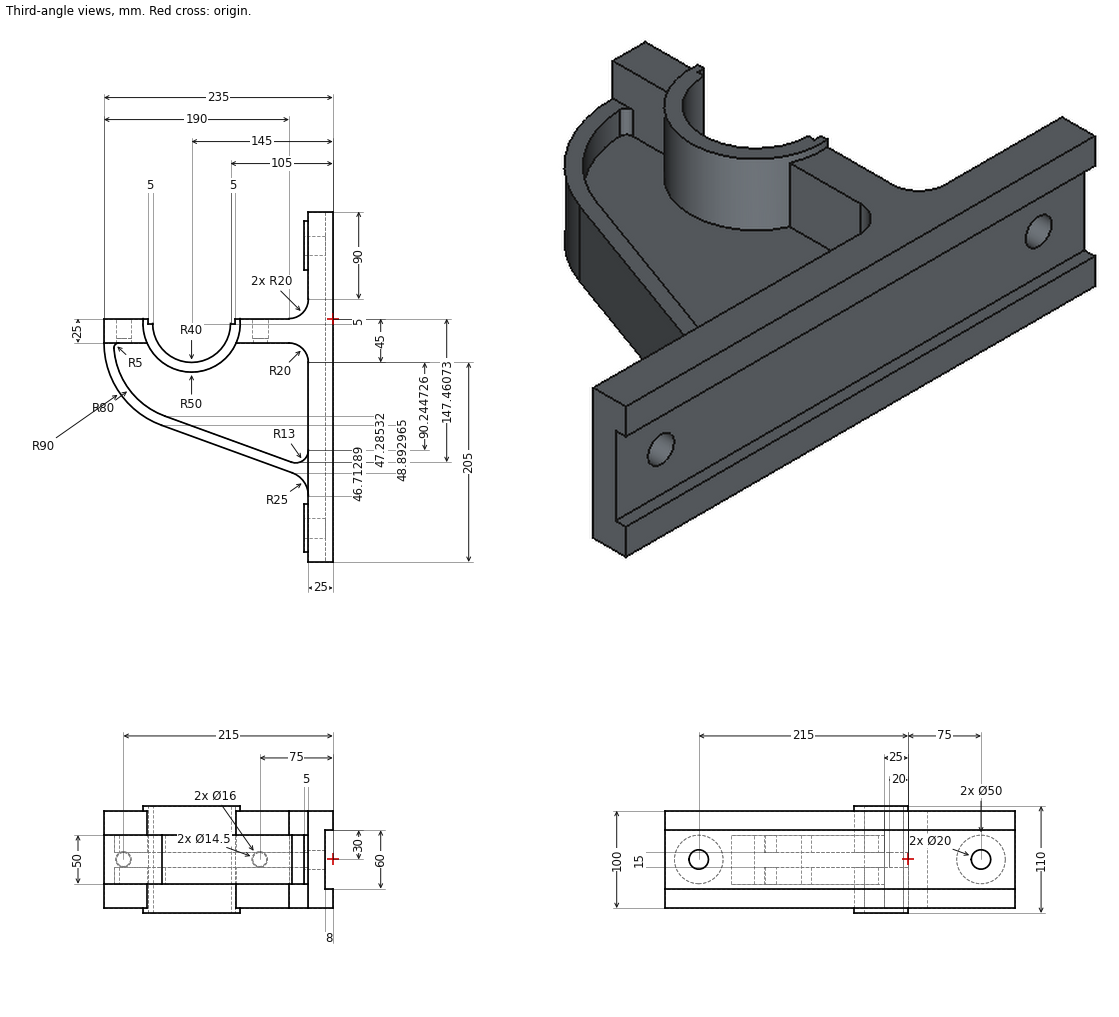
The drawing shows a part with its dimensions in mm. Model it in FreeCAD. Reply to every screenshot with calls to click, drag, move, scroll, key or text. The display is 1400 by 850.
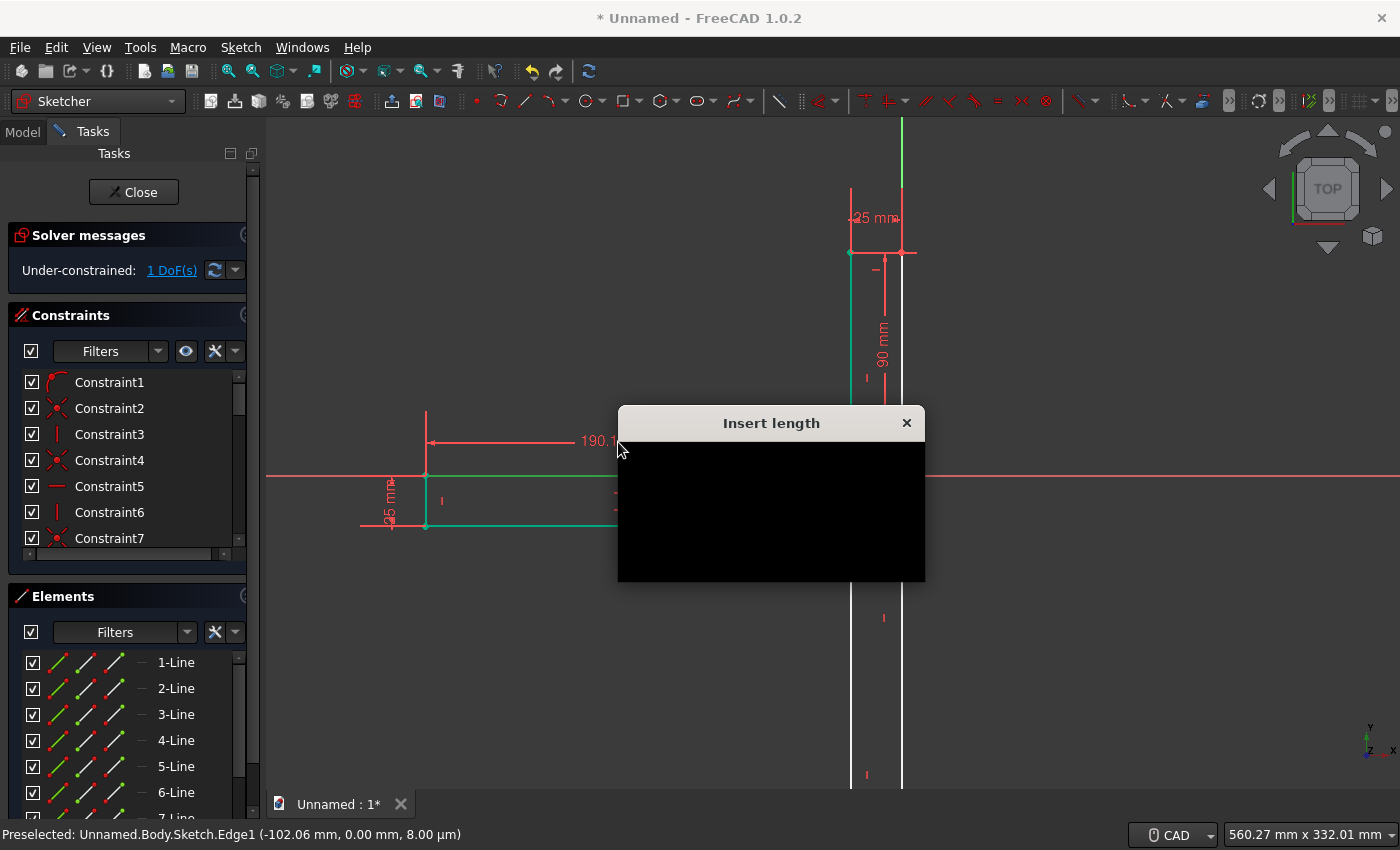
text(190)
key(Return)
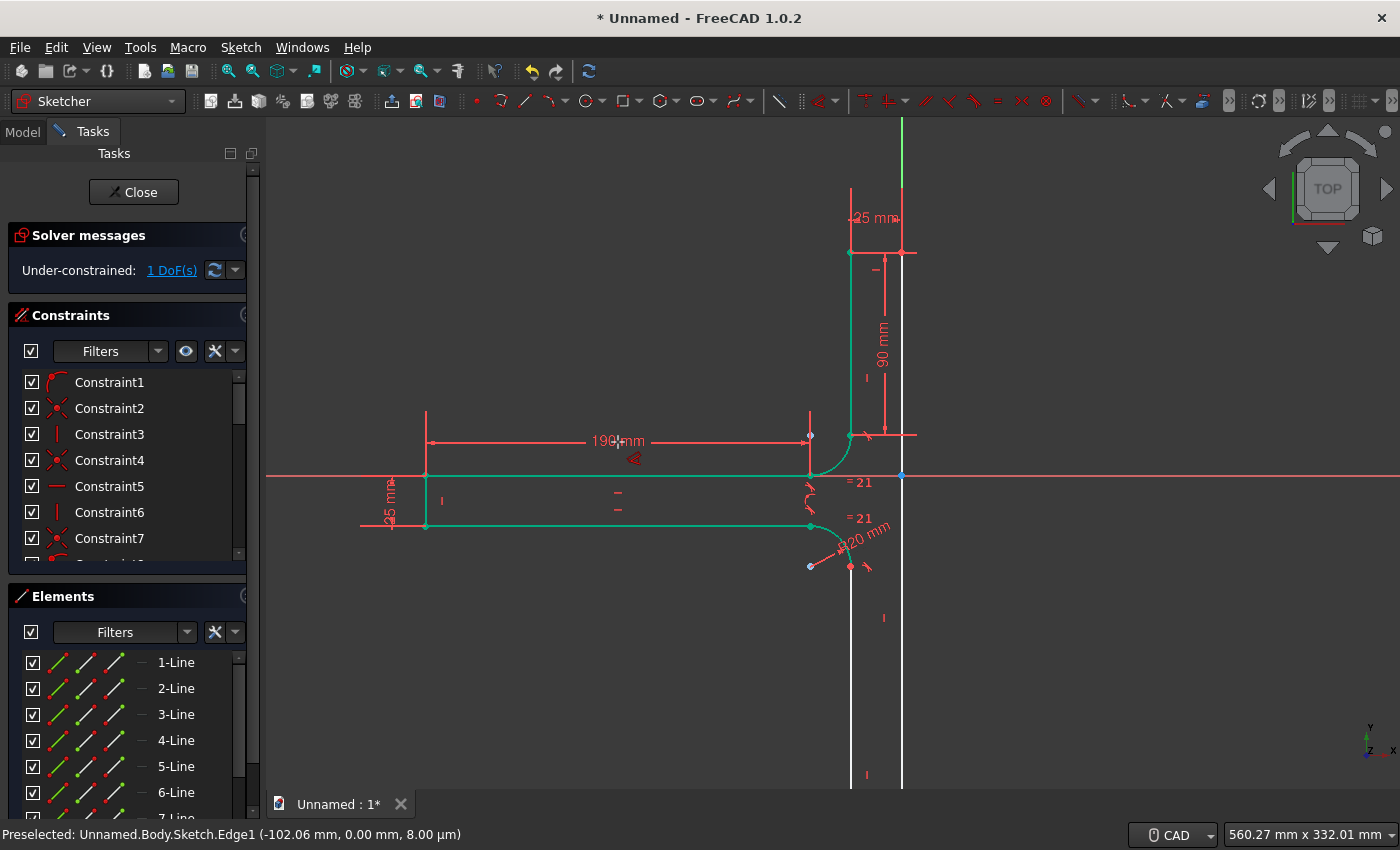
click(851, 691)
click(885, 664)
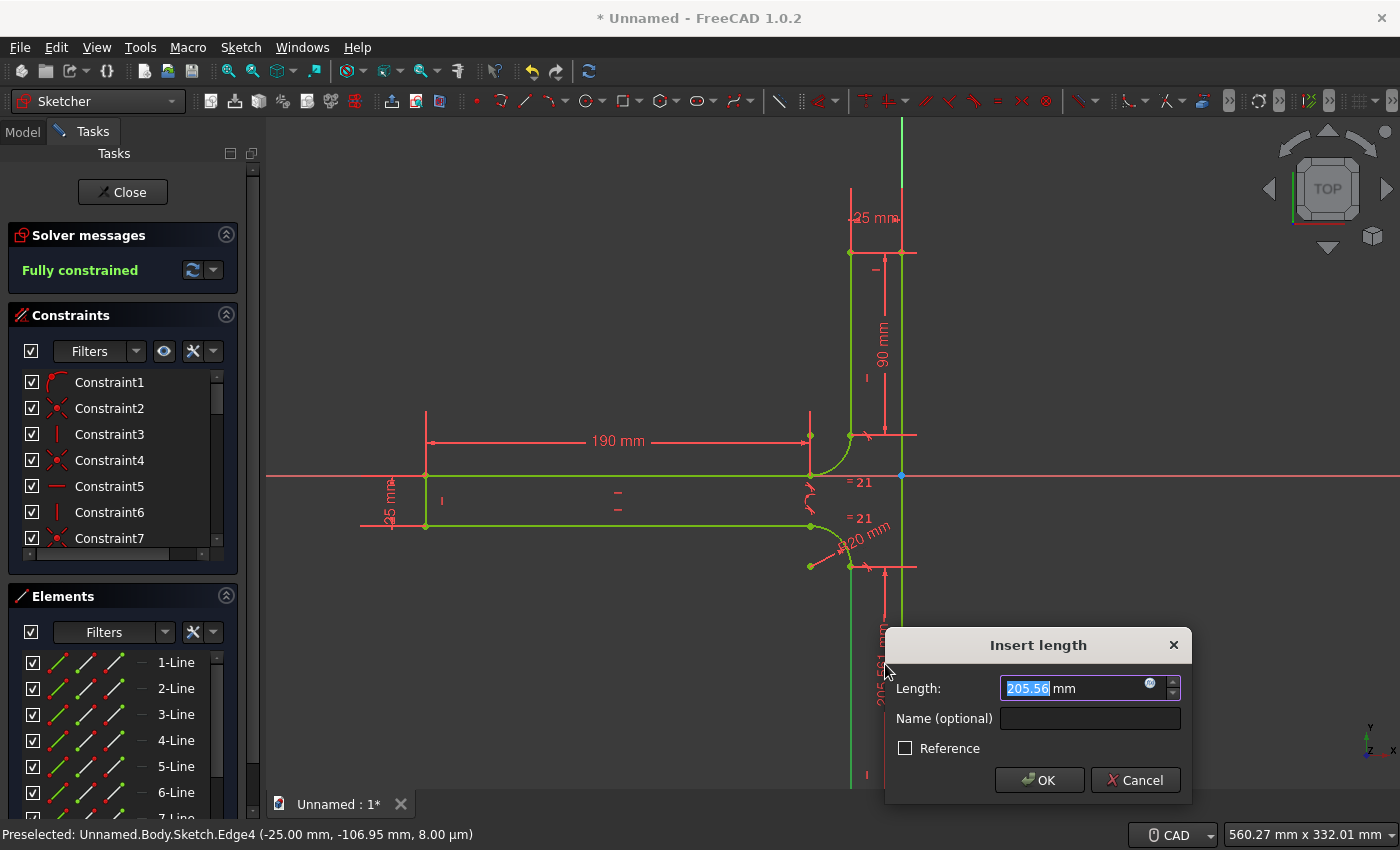
text(205)
key(Return)
key(Escape)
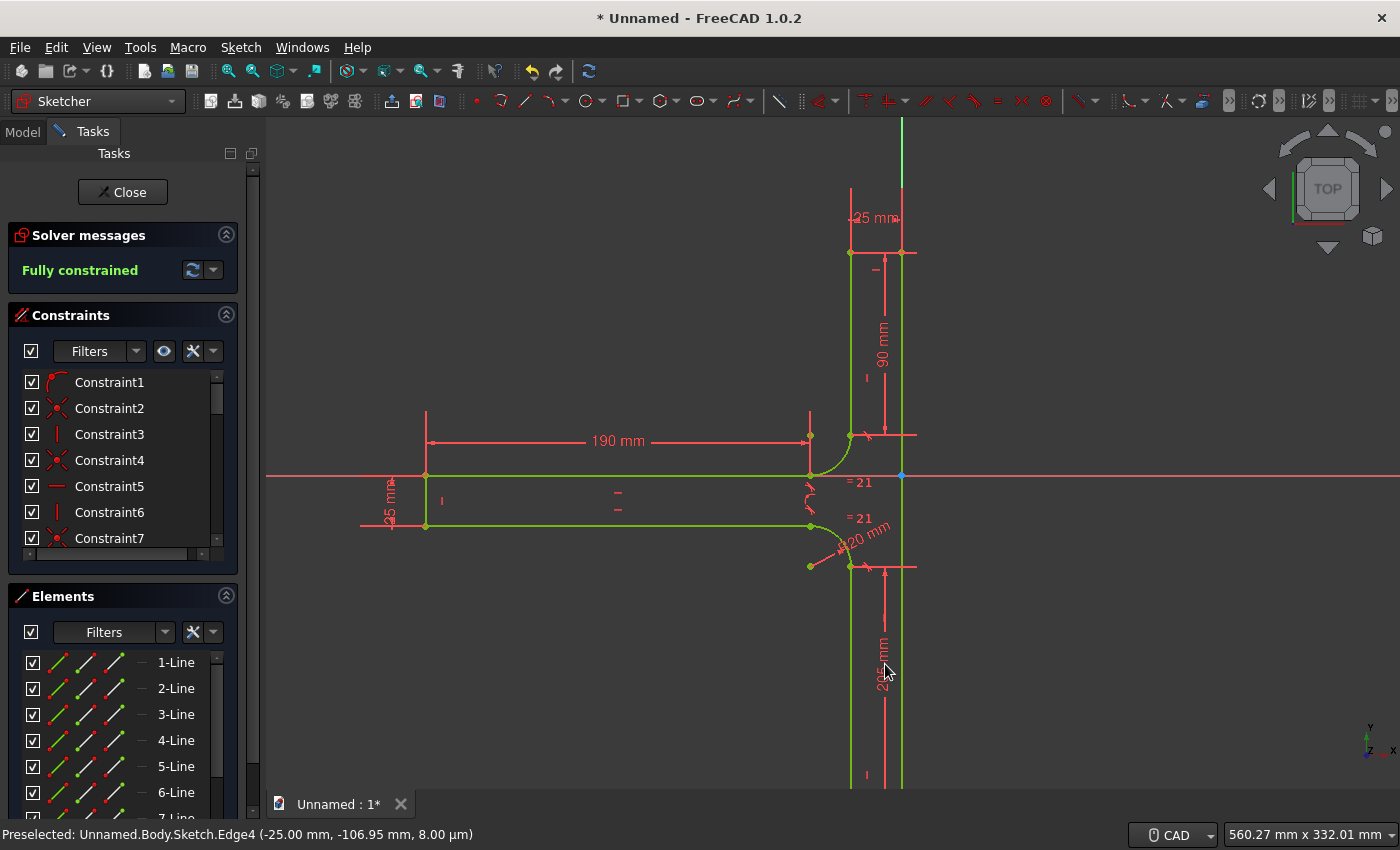
click(123, 192)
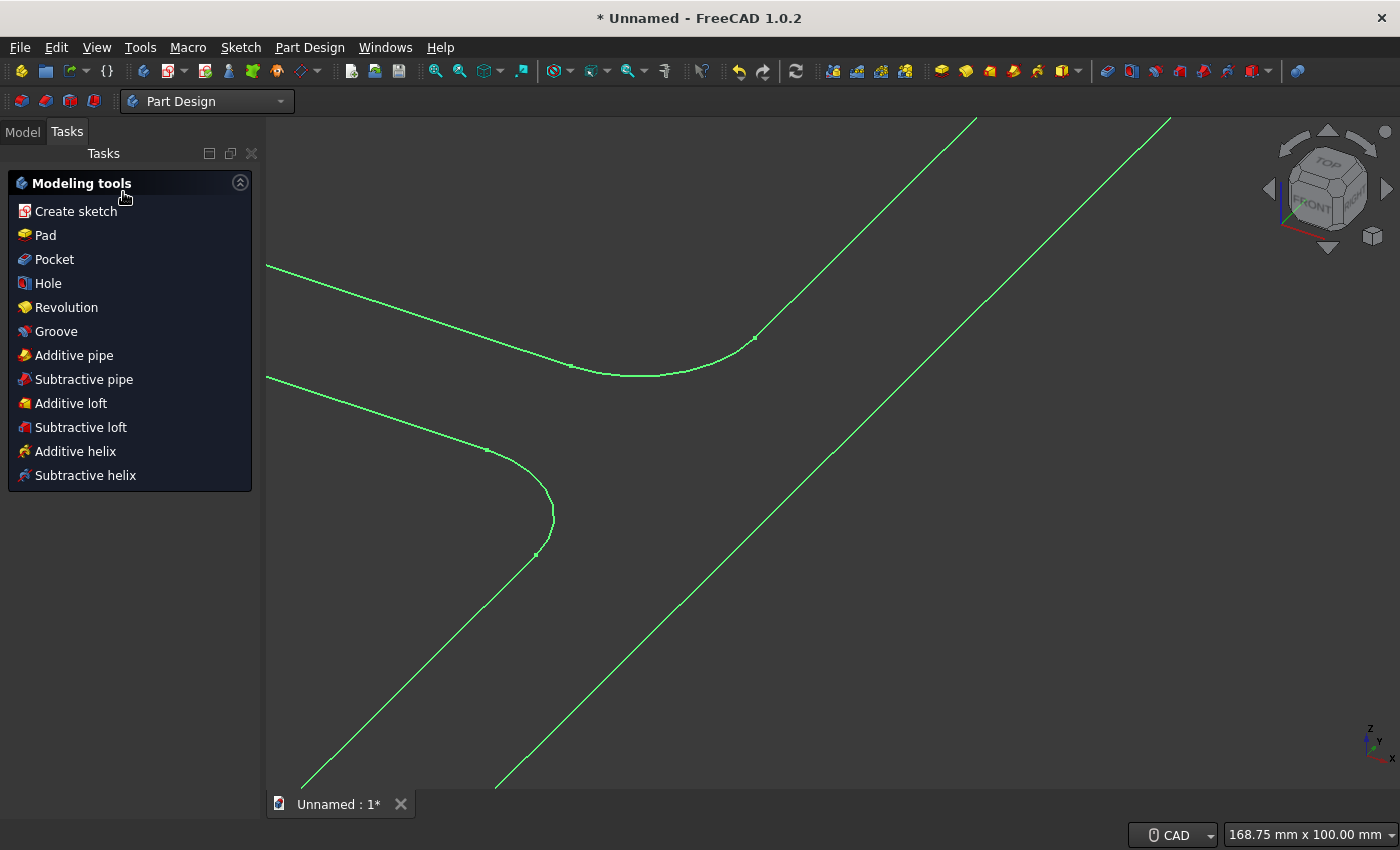
click(942, 72)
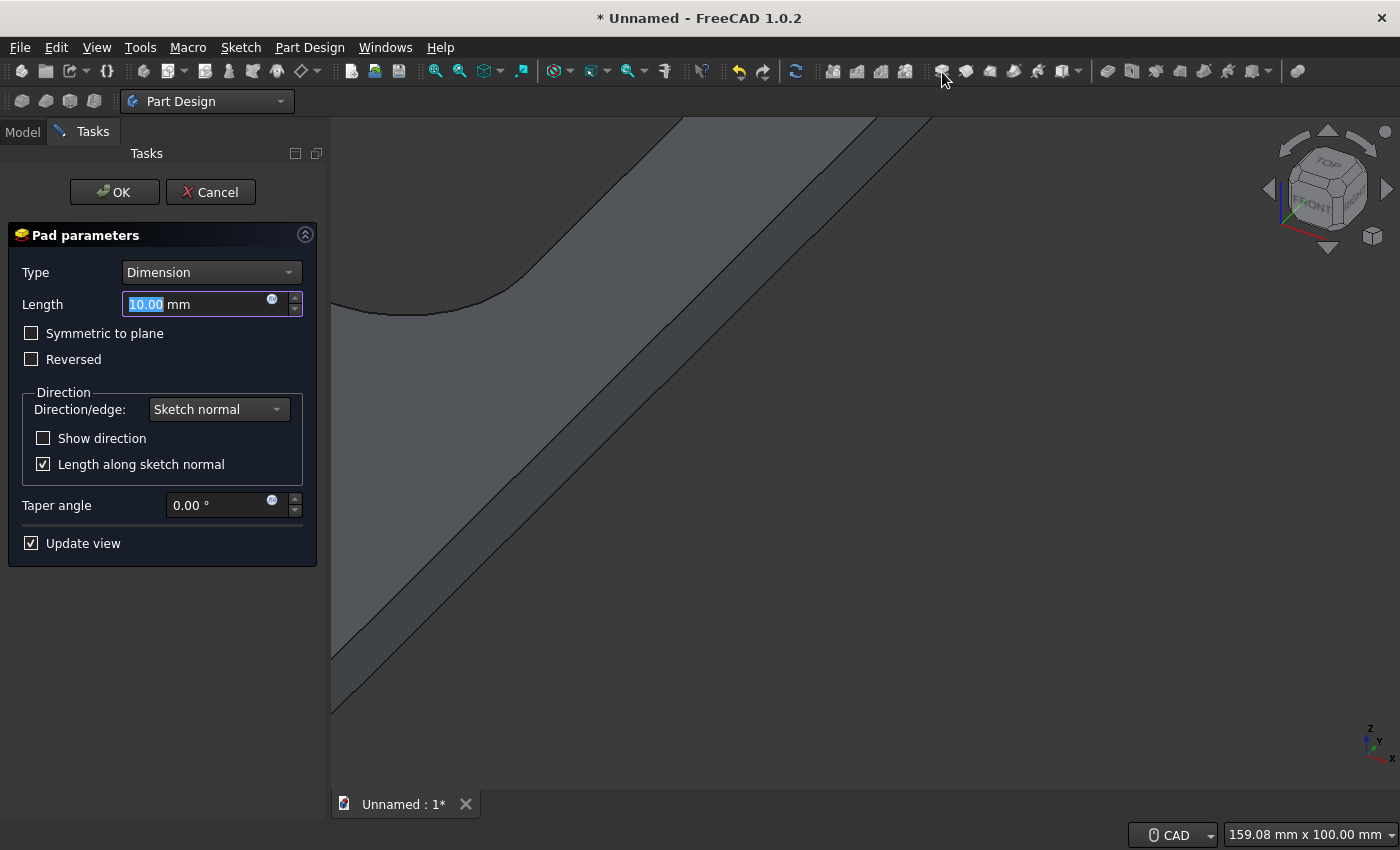
text(100)
key(Tab)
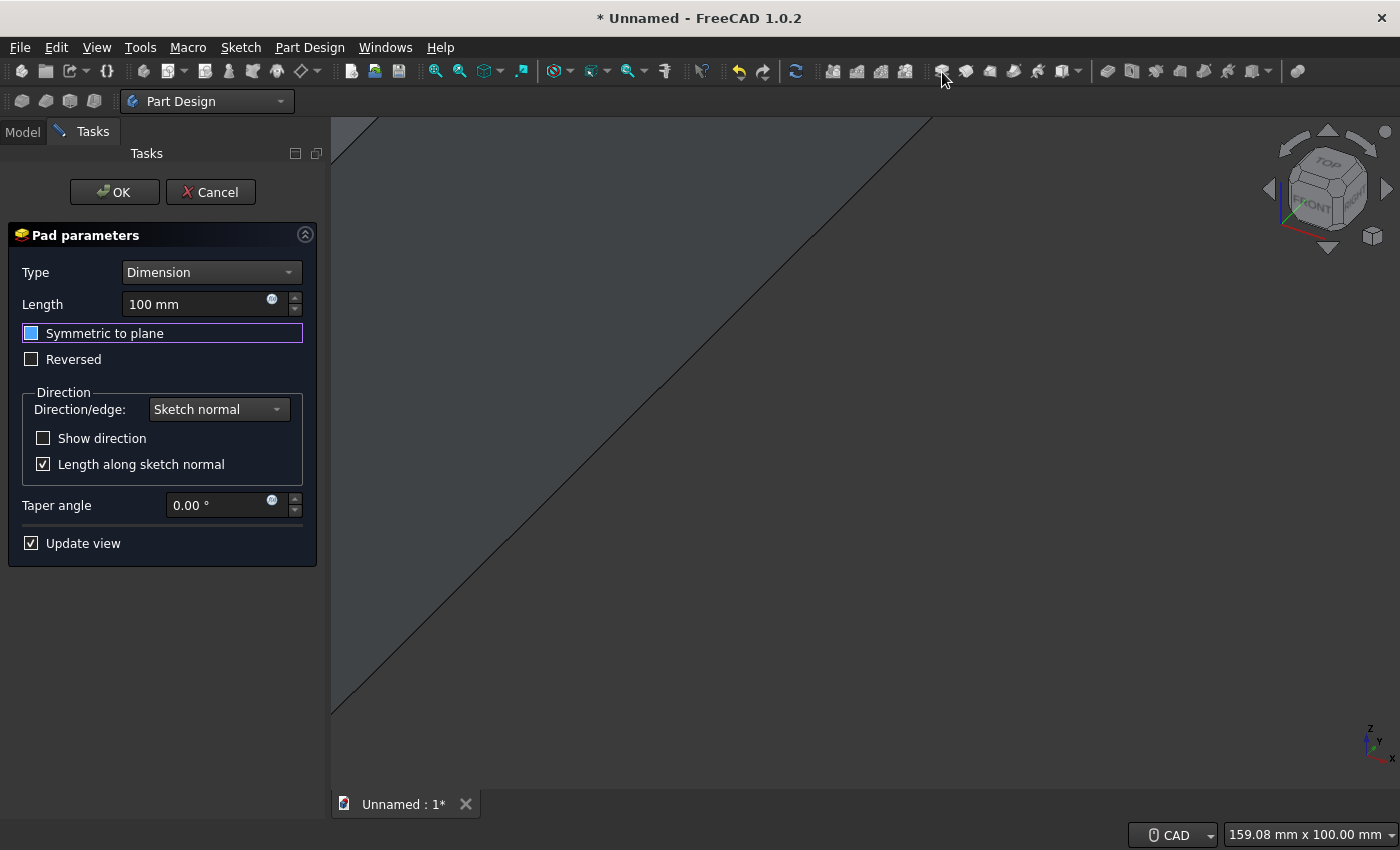
click(30, 333)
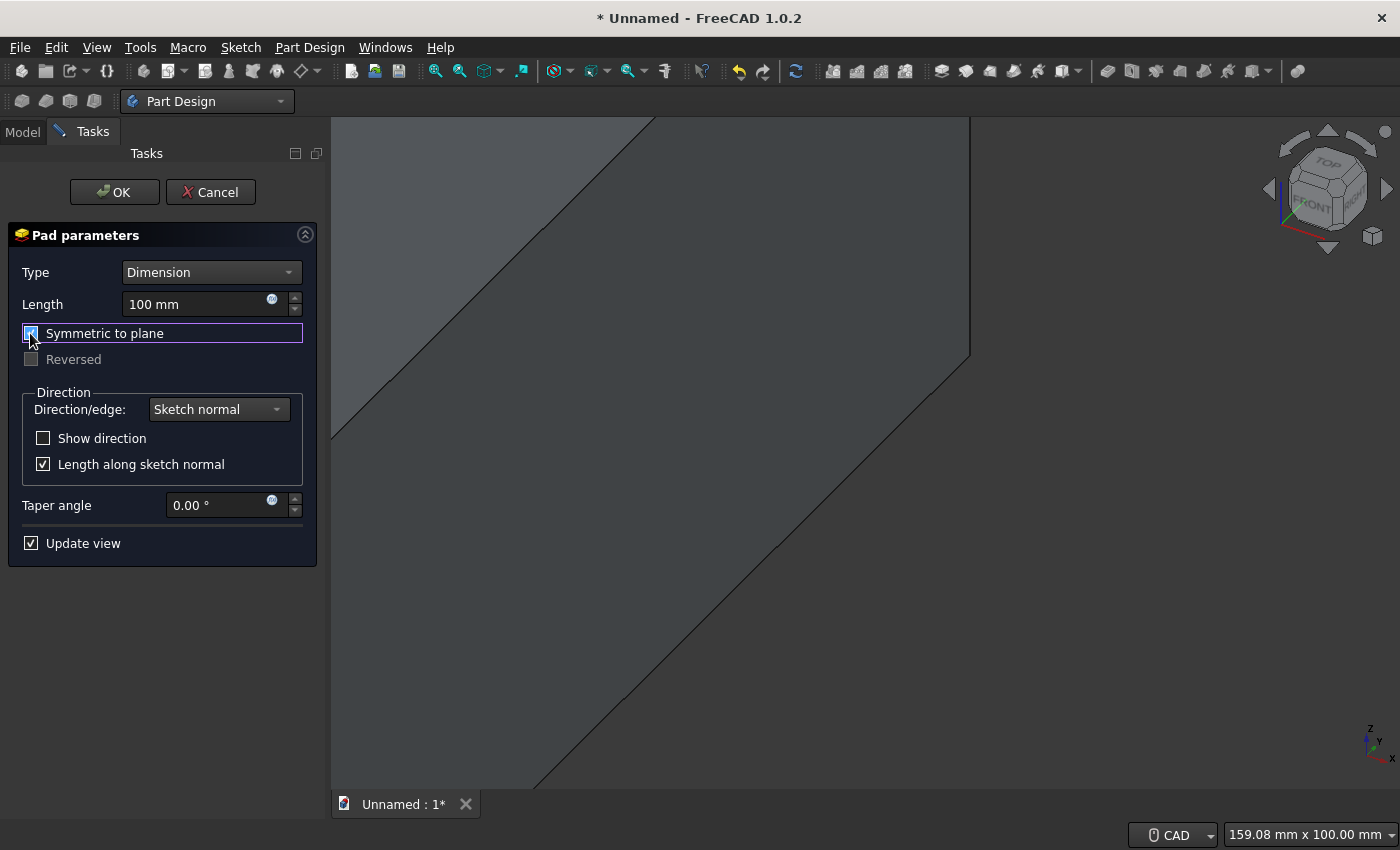
click(115, 192)